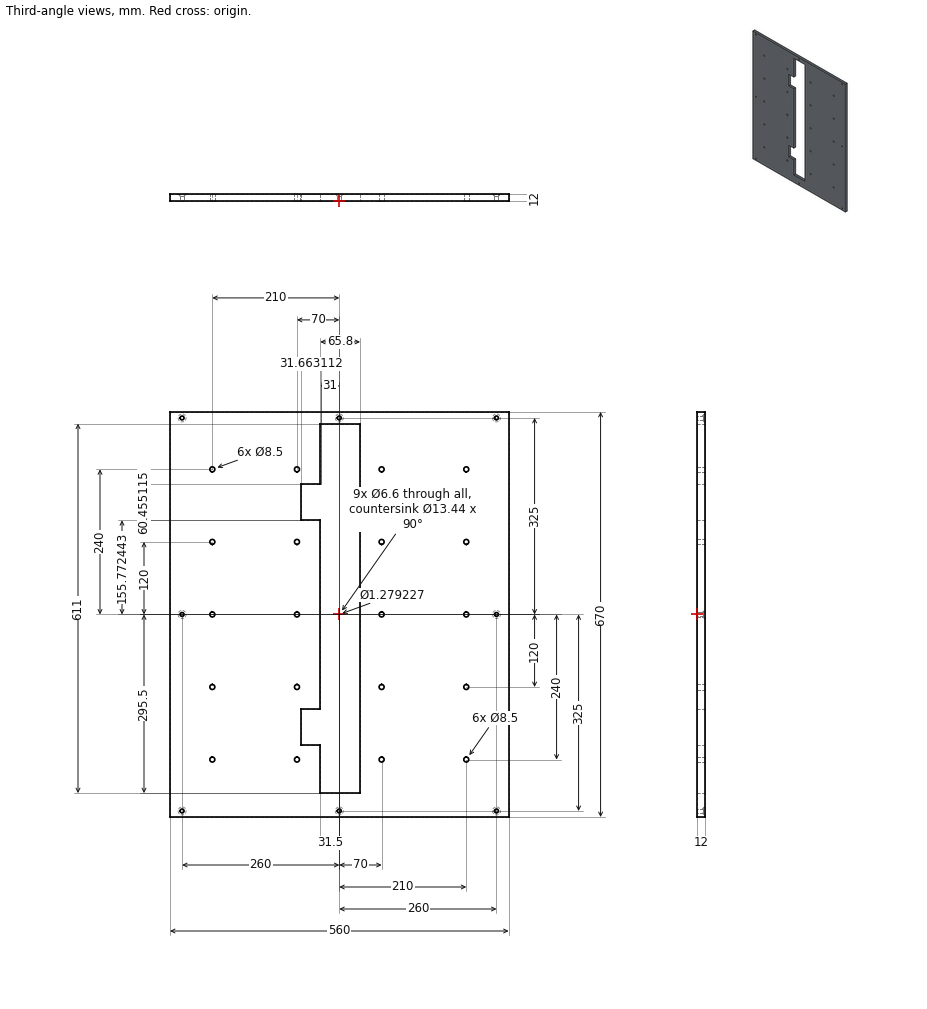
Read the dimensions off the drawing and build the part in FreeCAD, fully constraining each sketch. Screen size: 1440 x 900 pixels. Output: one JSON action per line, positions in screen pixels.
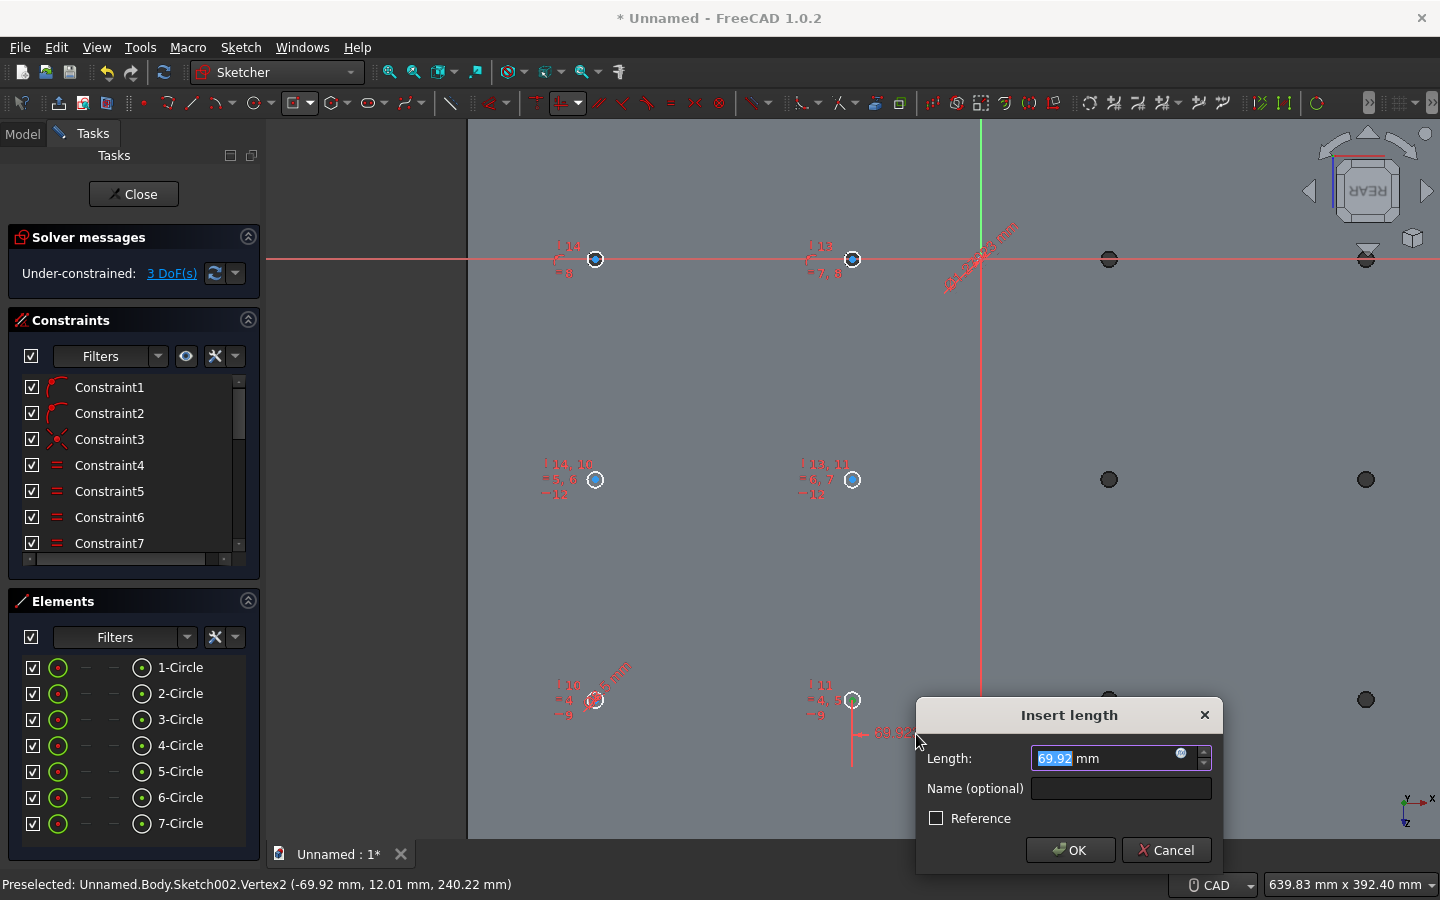
{"action": "type", "text": "70"}
{"action": "key", "text": "Return"}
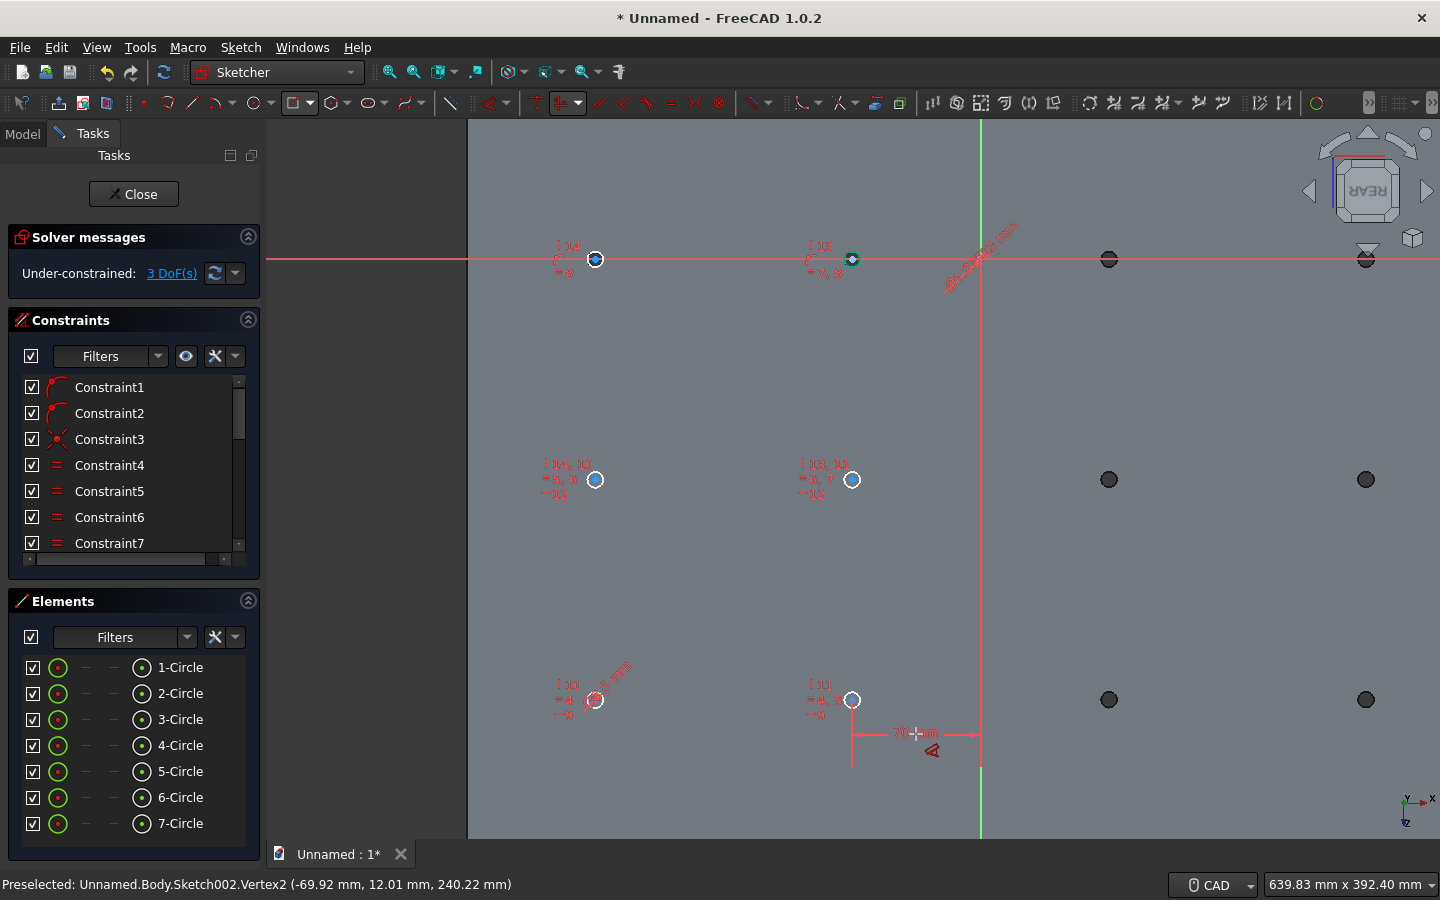
{"action": "left_click", "coordinate": [595, 700]}
{"action": "left_click", "coordinate": [788, 734]}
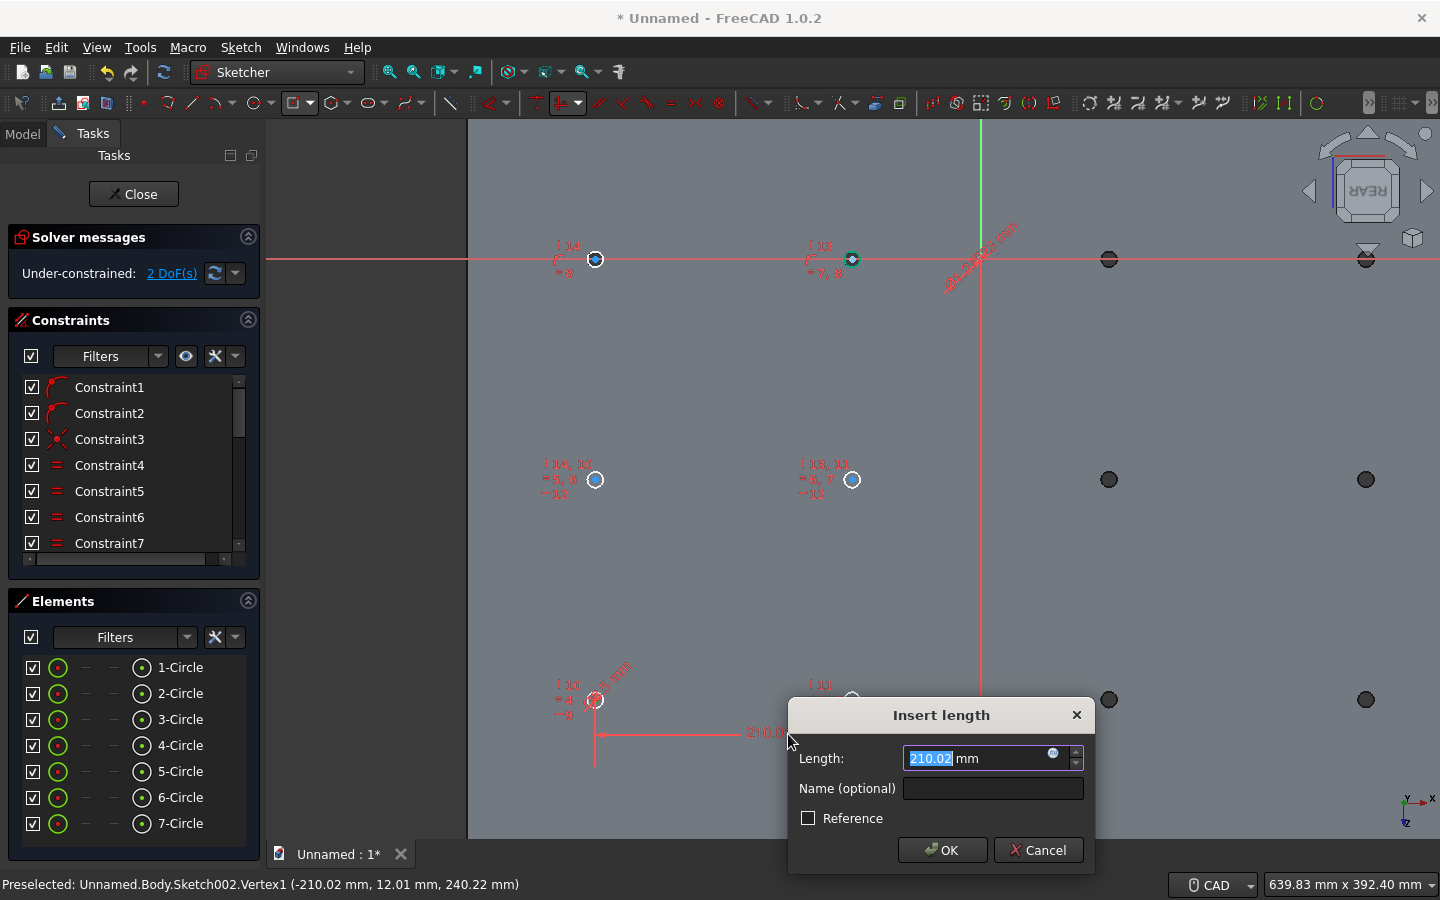
{"action": "type", "text": "210"}
{"action": "key", "text": "Return"}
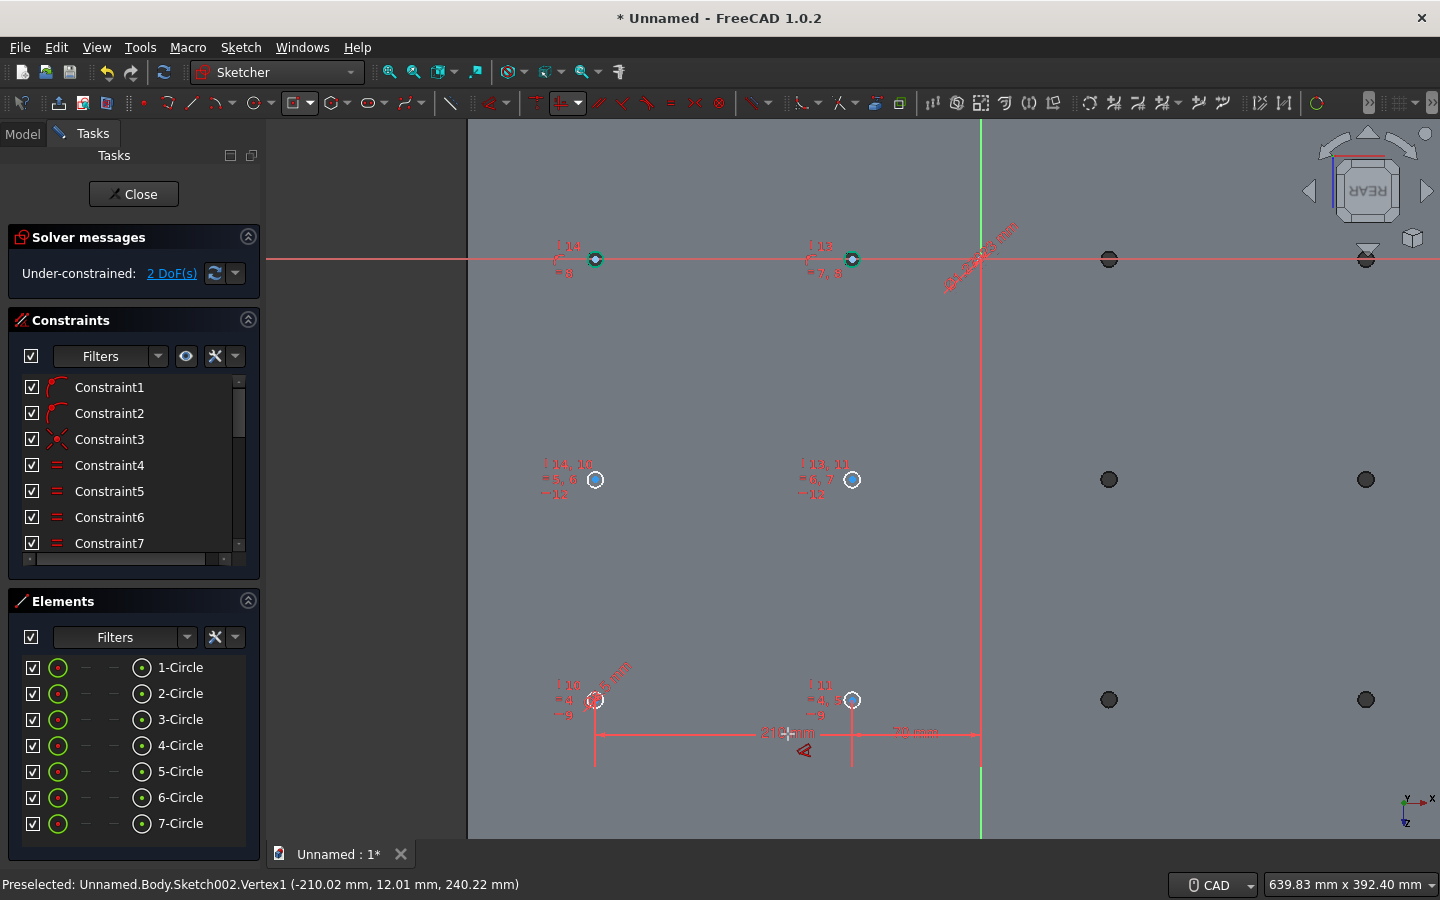
{"action": "left_click", "coordinate": [595, 700]}
{"action": "left_click", "coordinate": [1015, 480]}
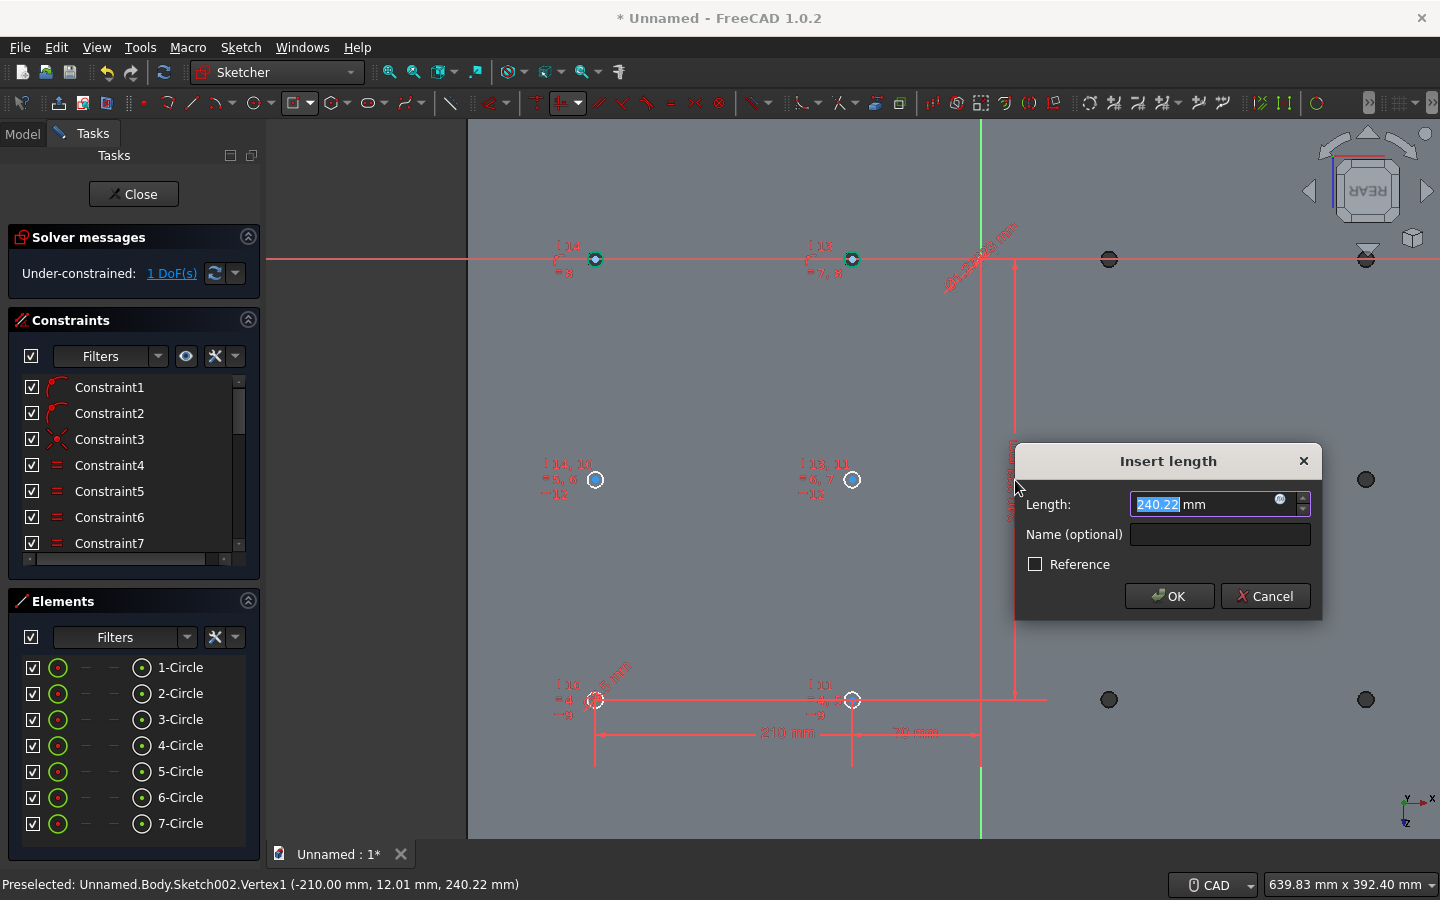
{"action": "type", "text": "240"}
{"action": "key", "text": "Return"}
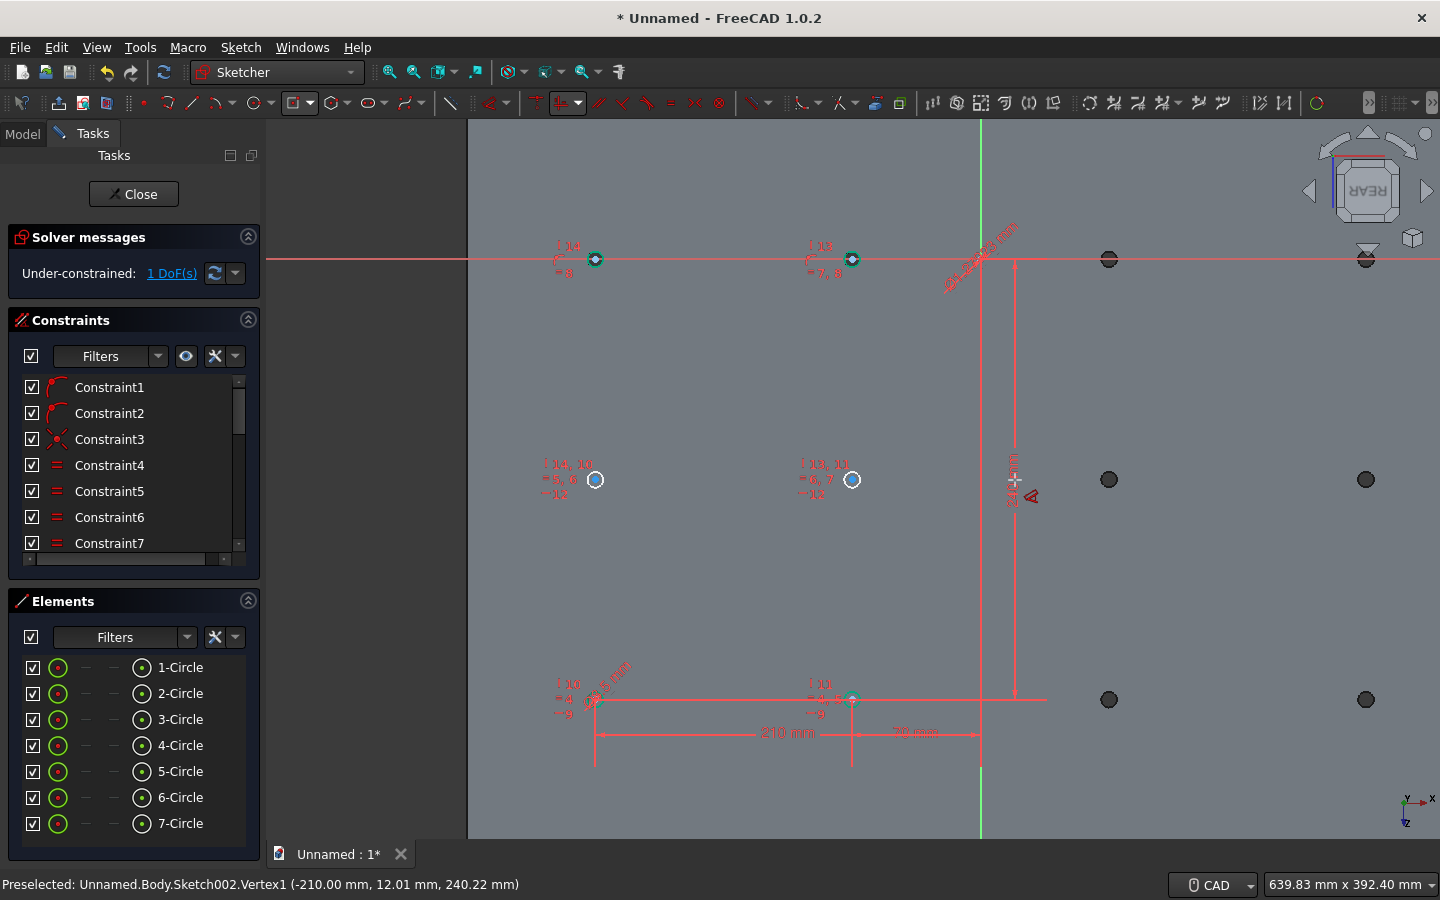
{"action": "left_click", "coordinate": [595, 480]}
{"action": "left_click", "coordinate": [1015, 370]}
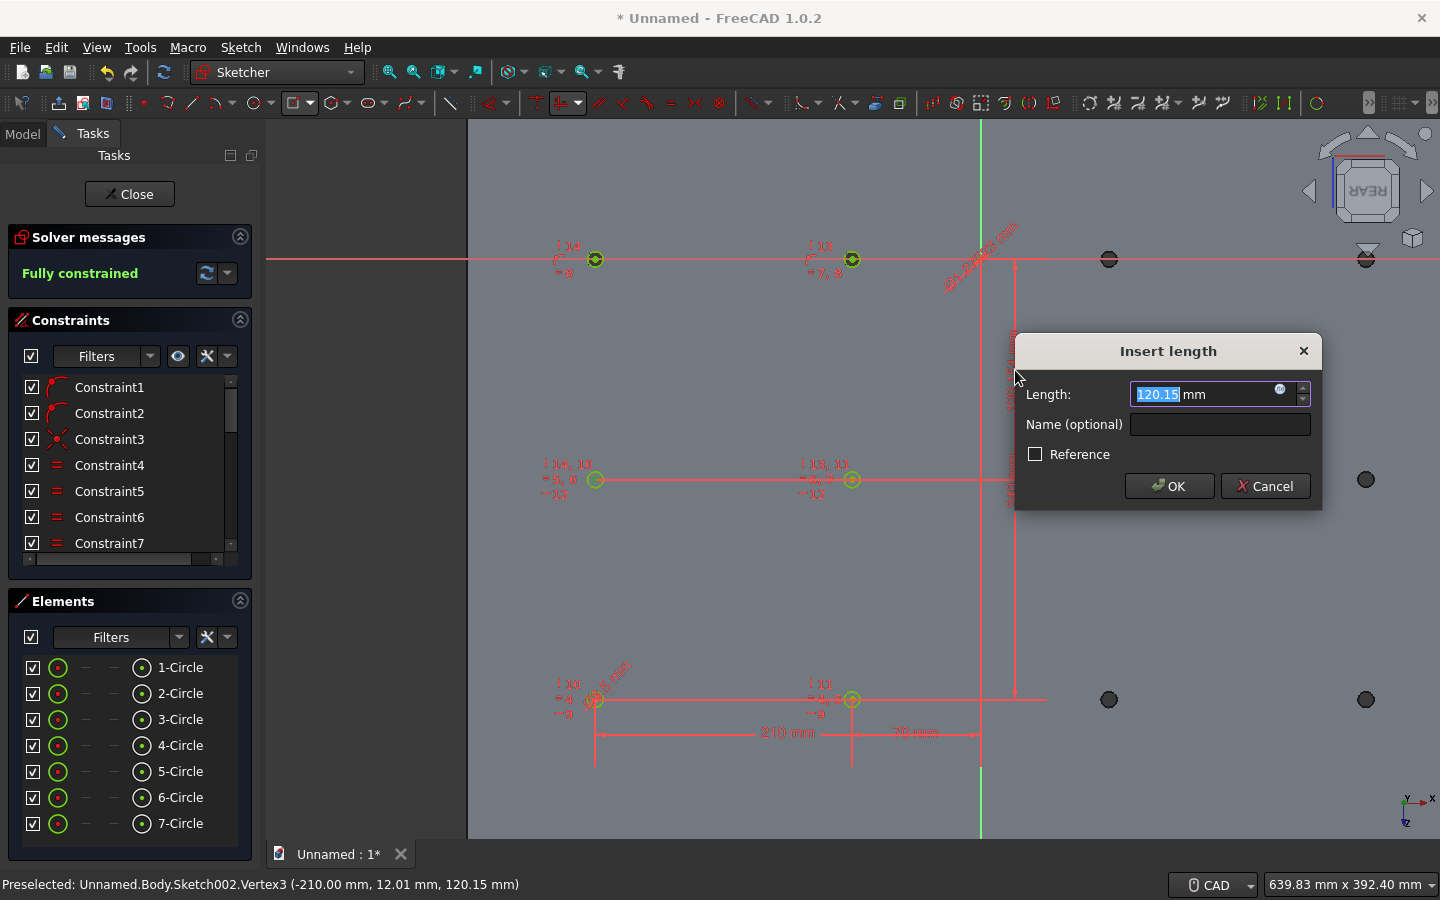
{"action": "type", "text": "120"}
{"action": "key", "text": "Return"}
{"action": "key", "text": "Escape"}